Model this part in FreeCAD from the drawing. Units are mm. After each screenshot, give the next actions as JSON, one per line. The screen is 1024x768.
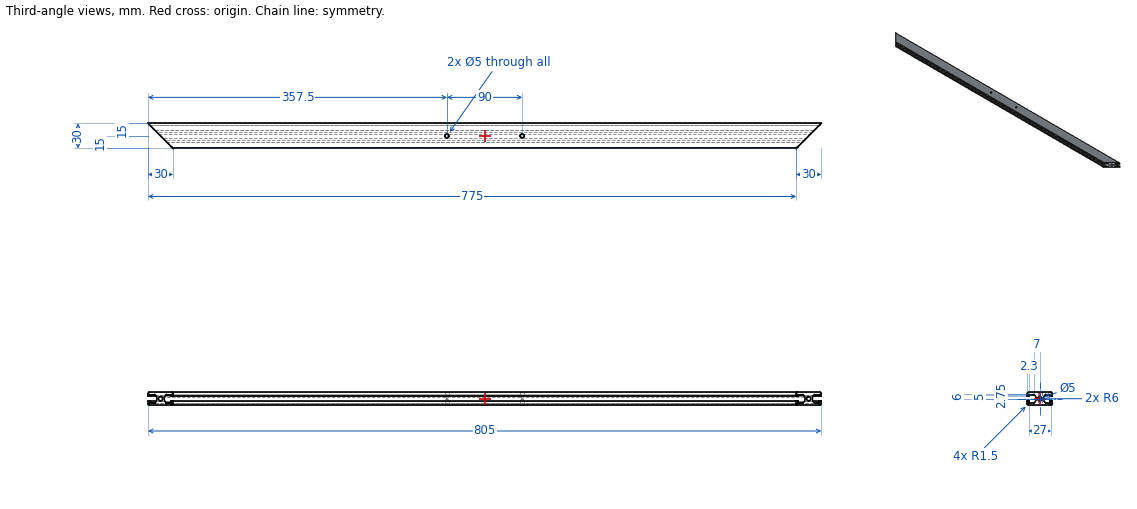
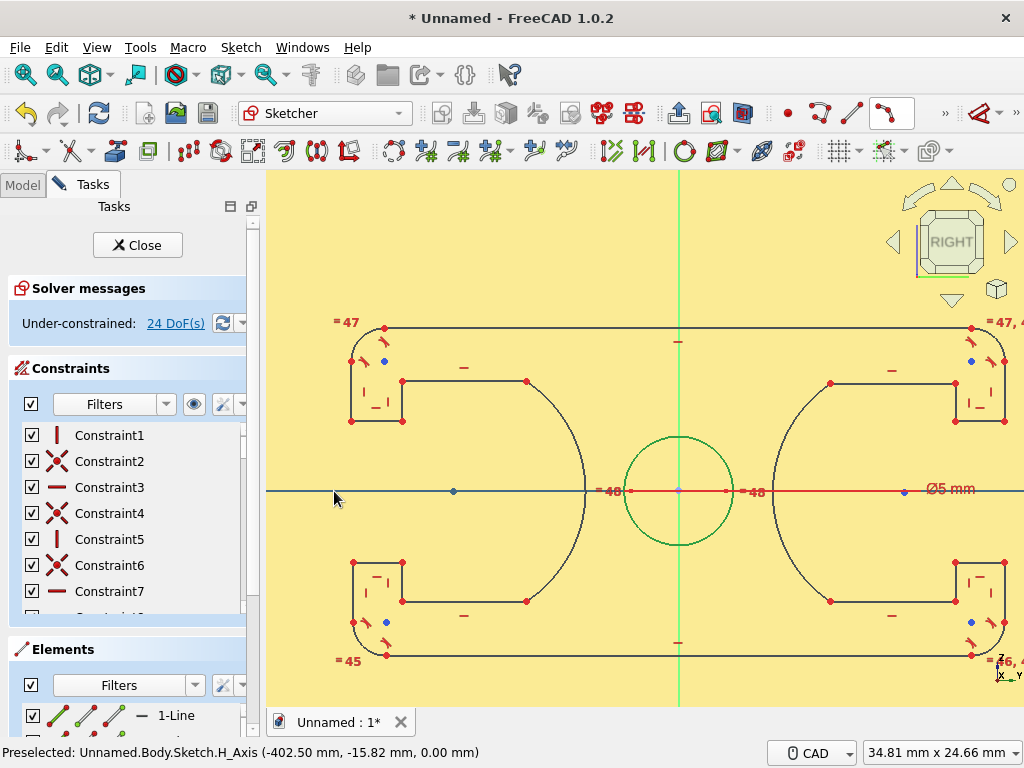
{"action": "key", "text": "c"}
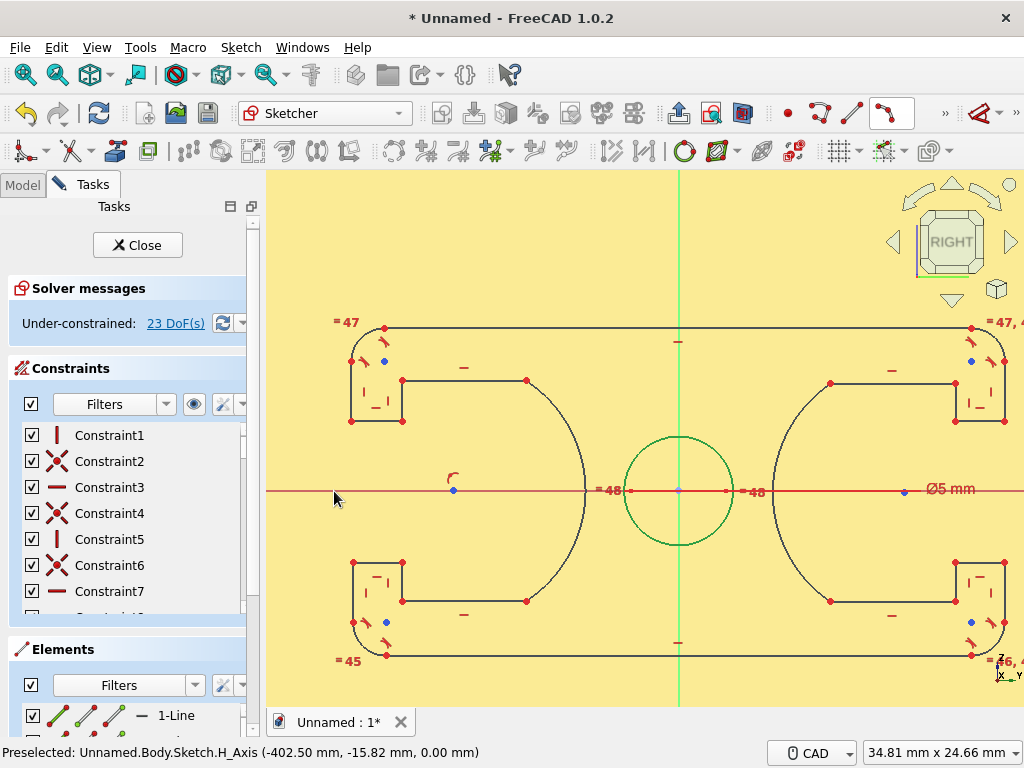
{"action": "scroll", "coordinate": [369, 332], "scroll_direction": "down", "scroll_amount": 2}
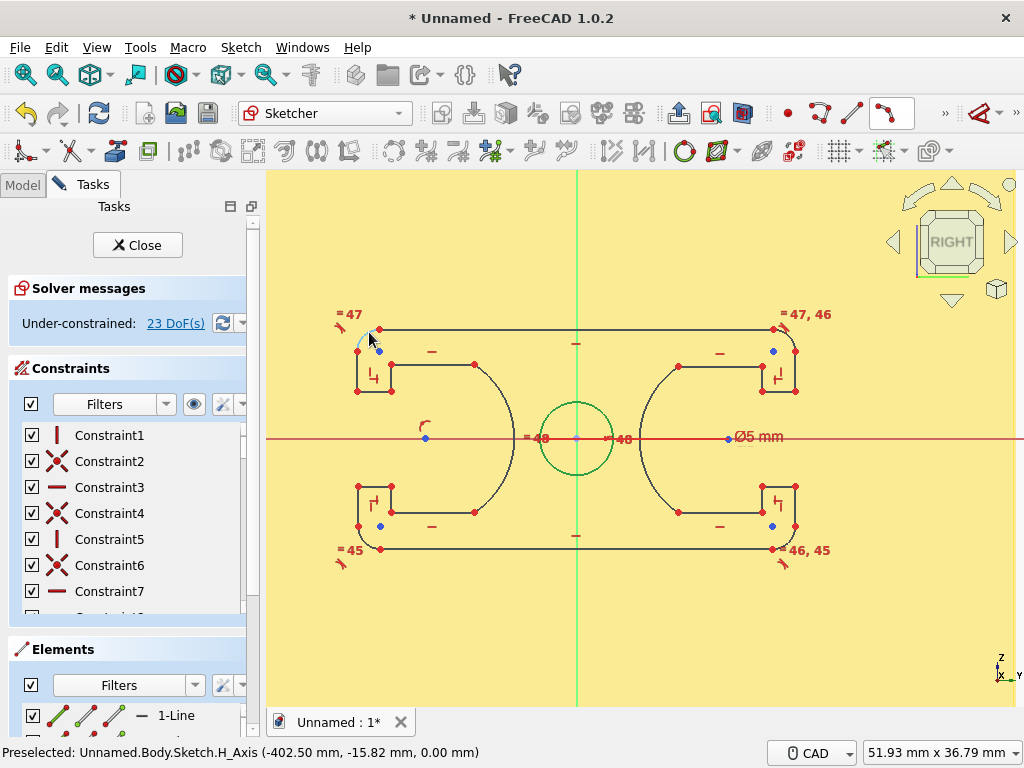
{"action": "left_click", "coordinate": [728, 440]}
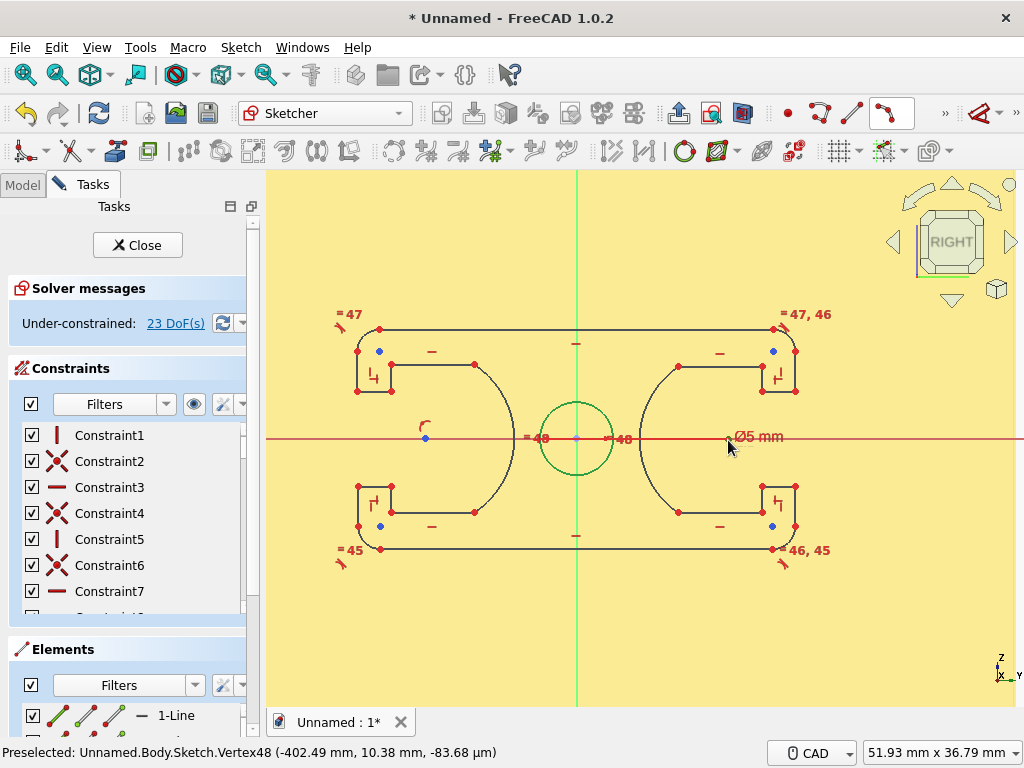
{"action": "left_click", "coordinate": [334, 439]}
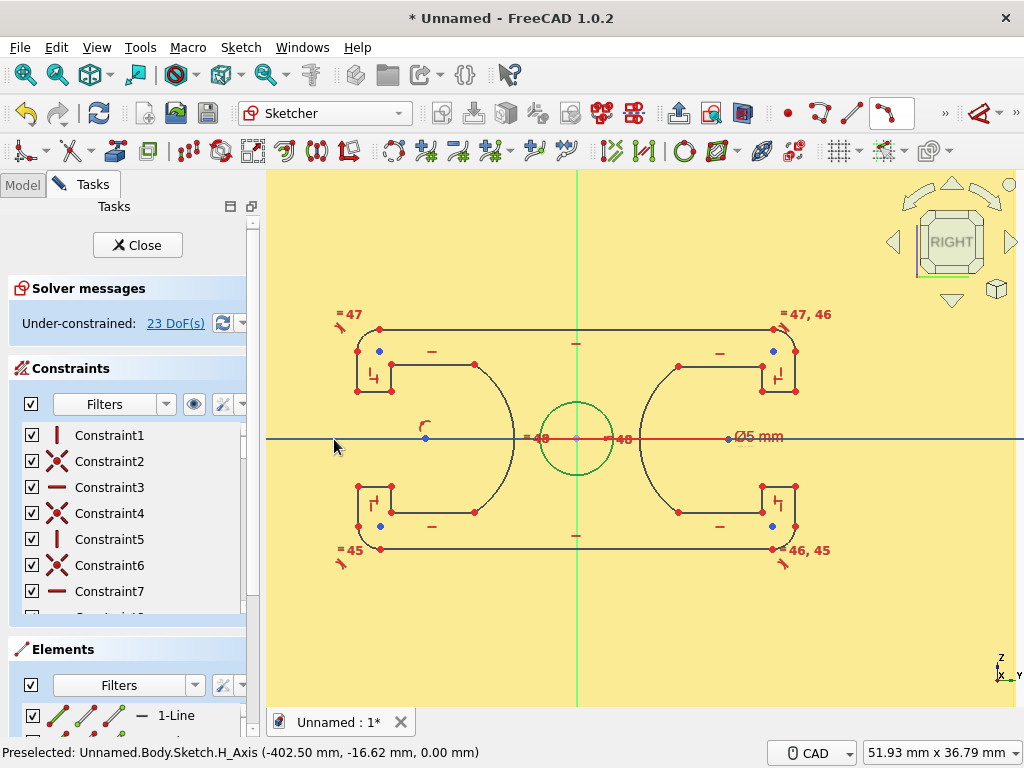
{"action": "key", "text": "c"}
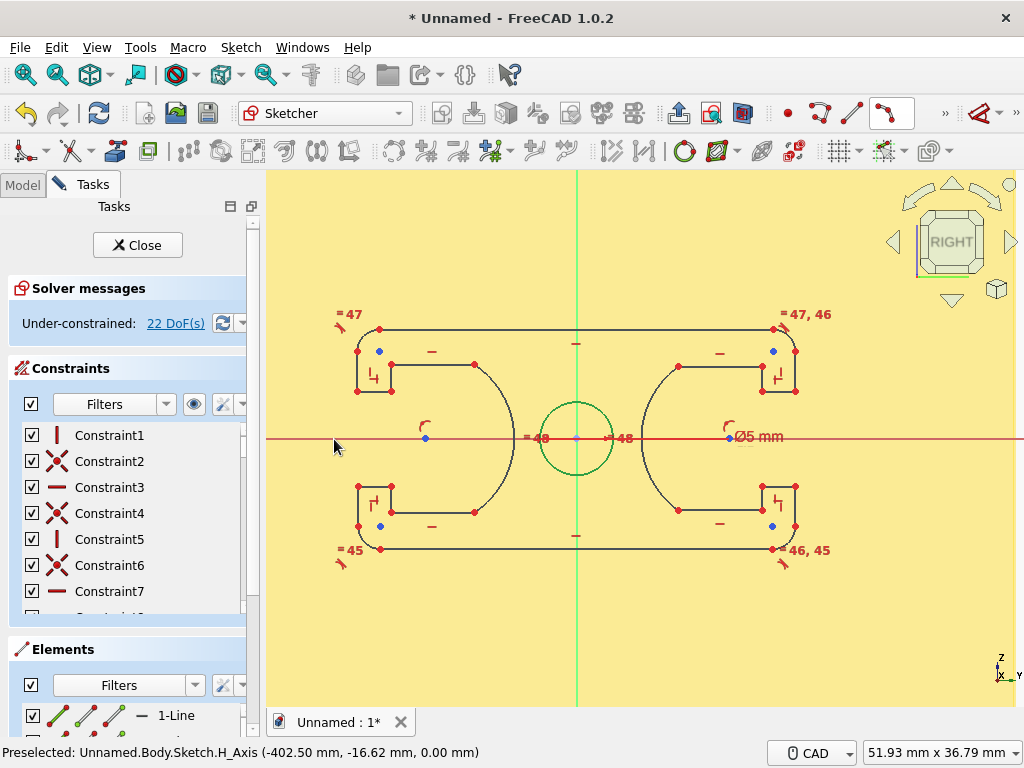
{"action": "left_click", "coordinate": [773, 527]}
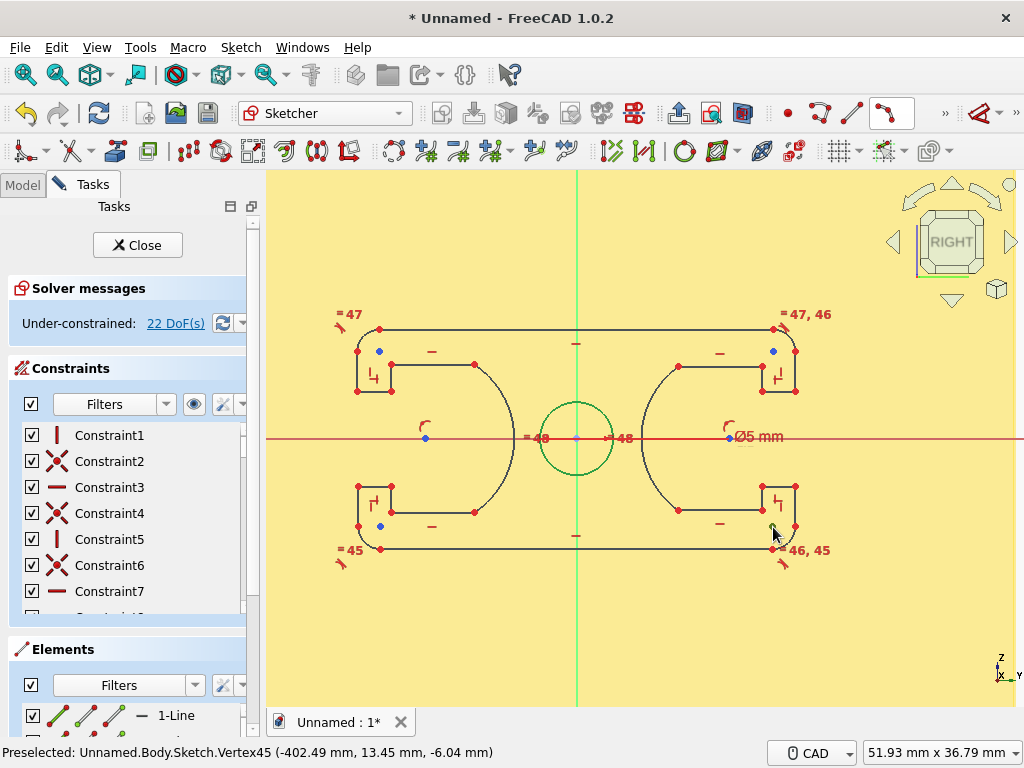
{"action": "left_click", "coordinate": [773, 352]}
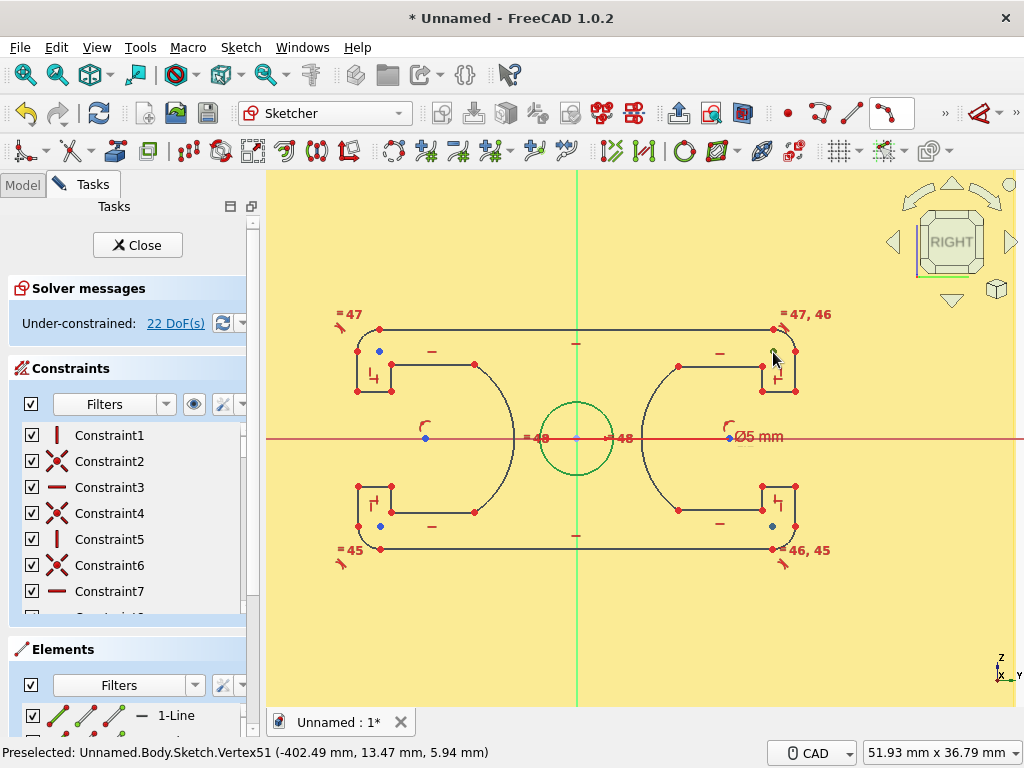
{"action": "left_click", "coordinate": [334, 439]}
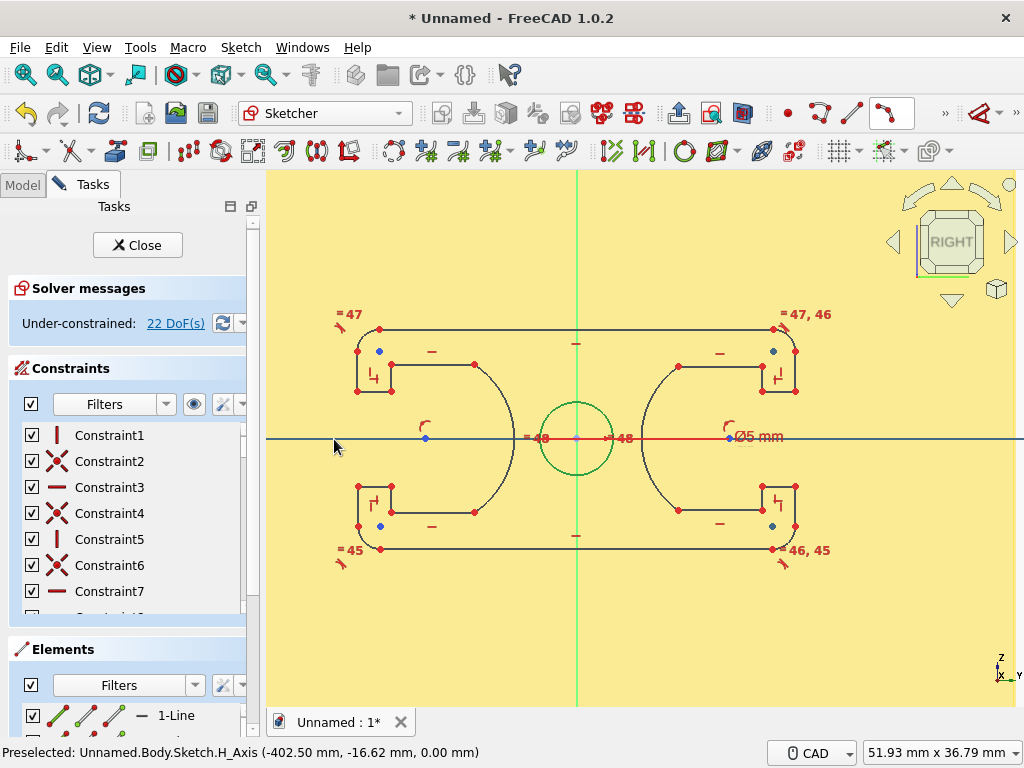
{"action": "key", "text": "s"}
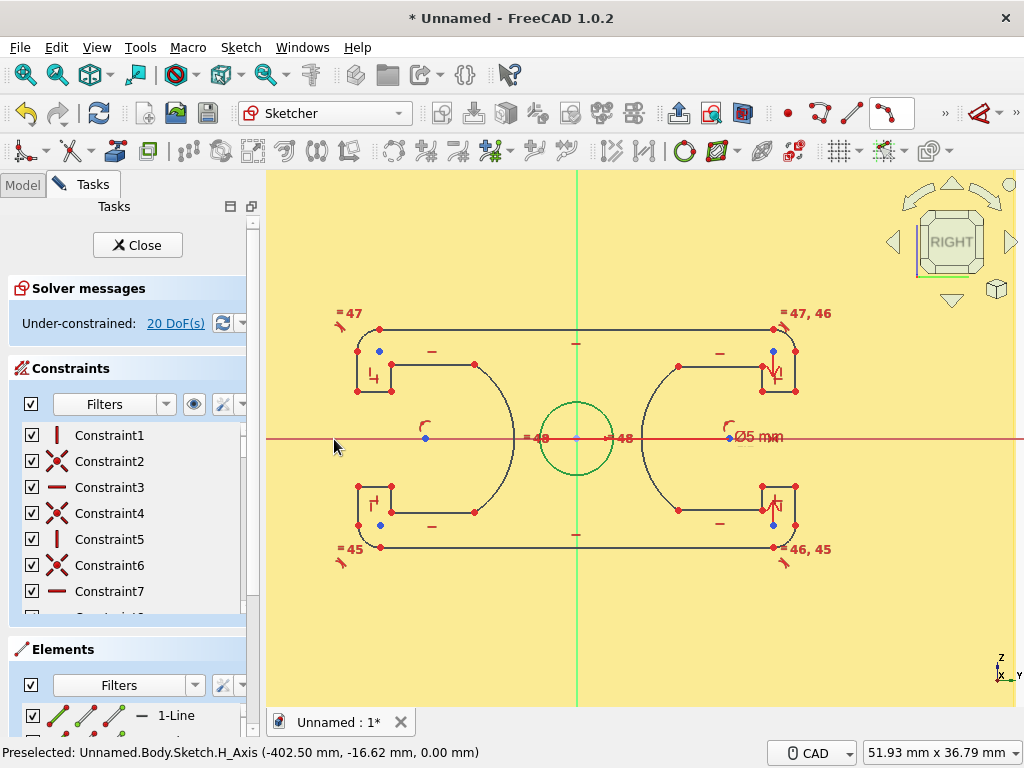
{"action": "left_click", "coordinate": [391, 365]}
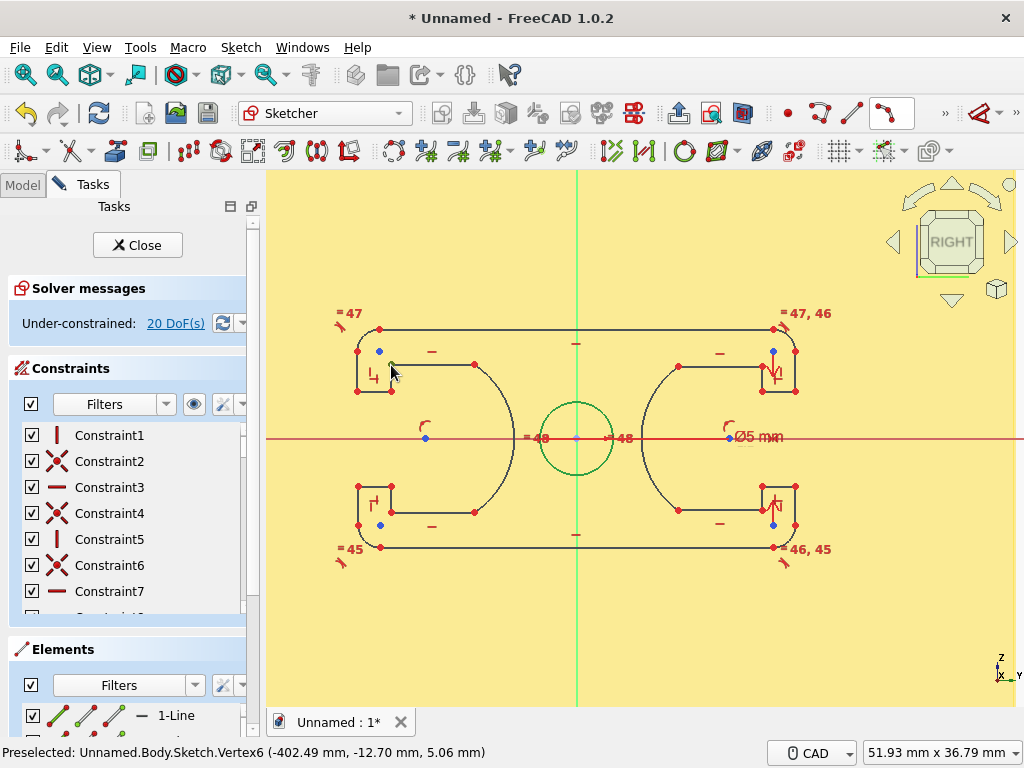
{"action": "left_click", "coordinate": [391, 513]}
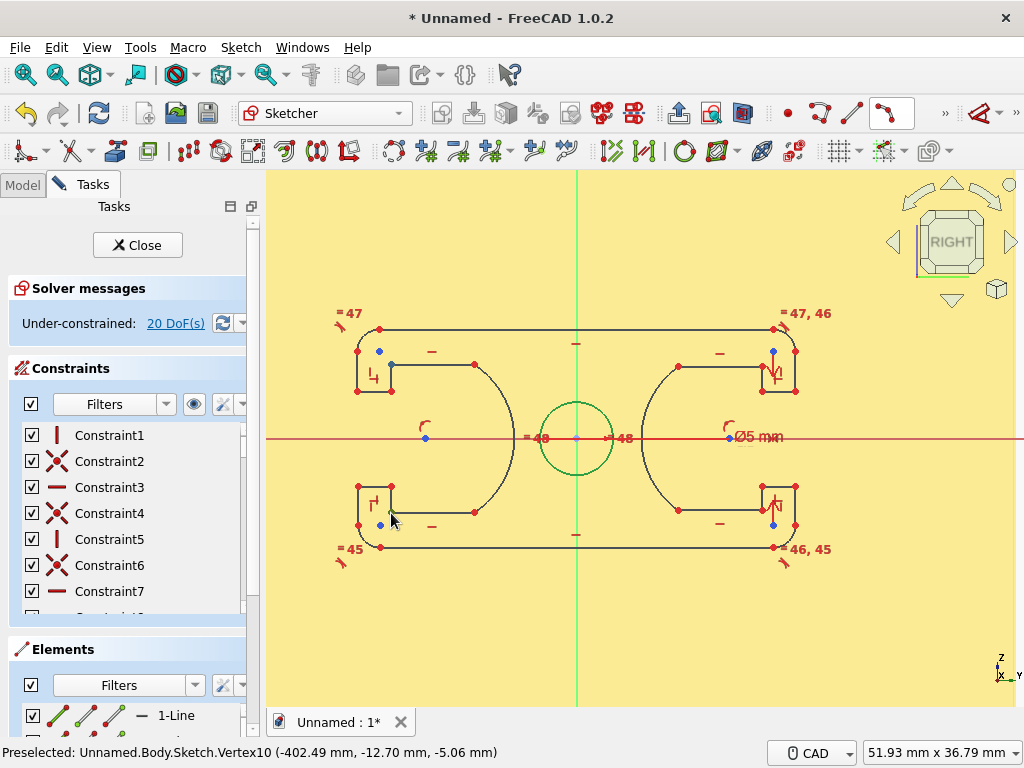
{"action": "left_click", "coordinate": [334, 439]}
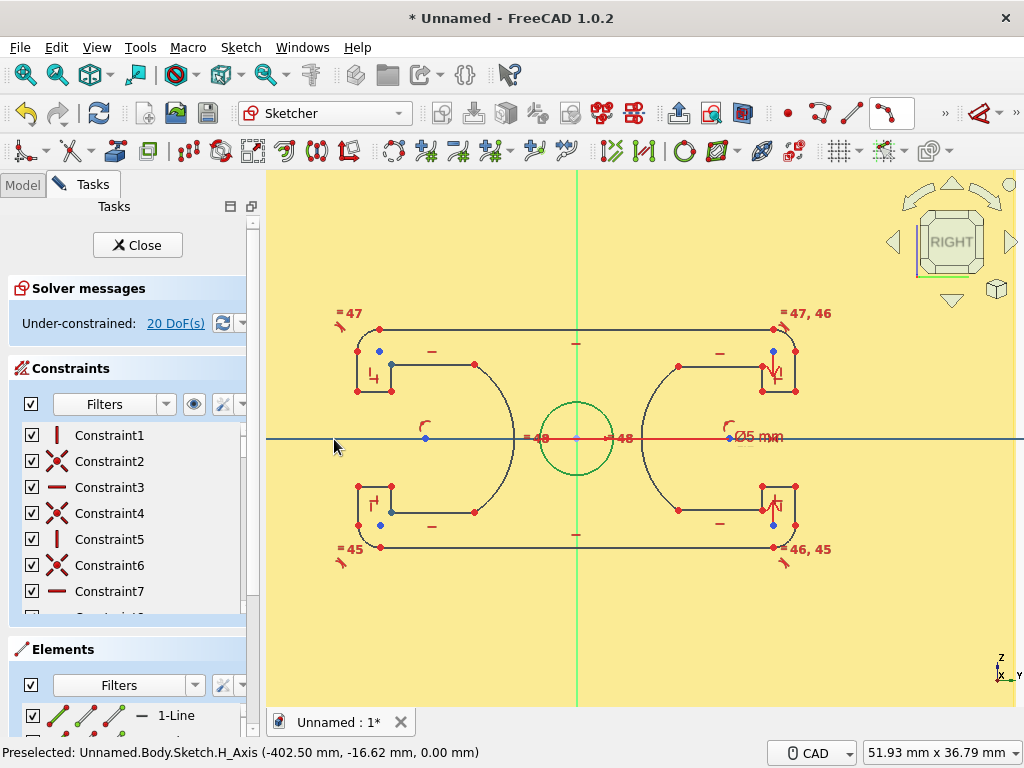
{"action": "key", "text": "s"}